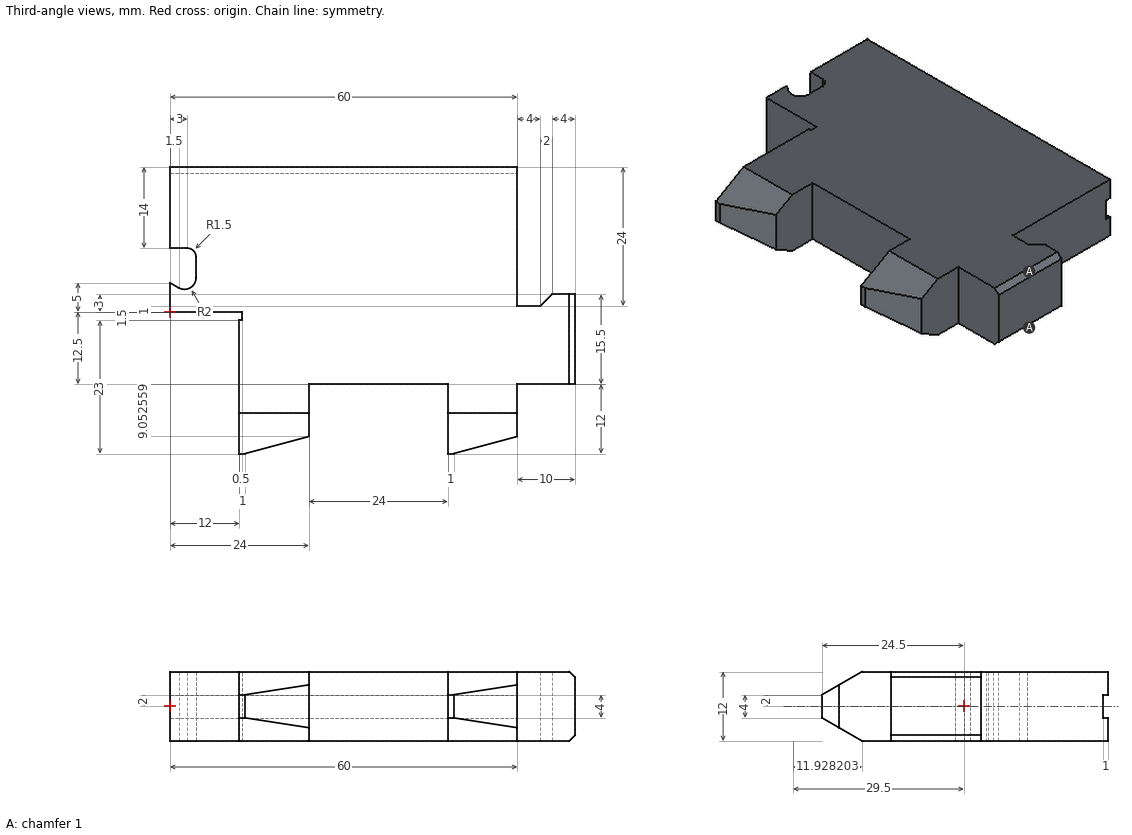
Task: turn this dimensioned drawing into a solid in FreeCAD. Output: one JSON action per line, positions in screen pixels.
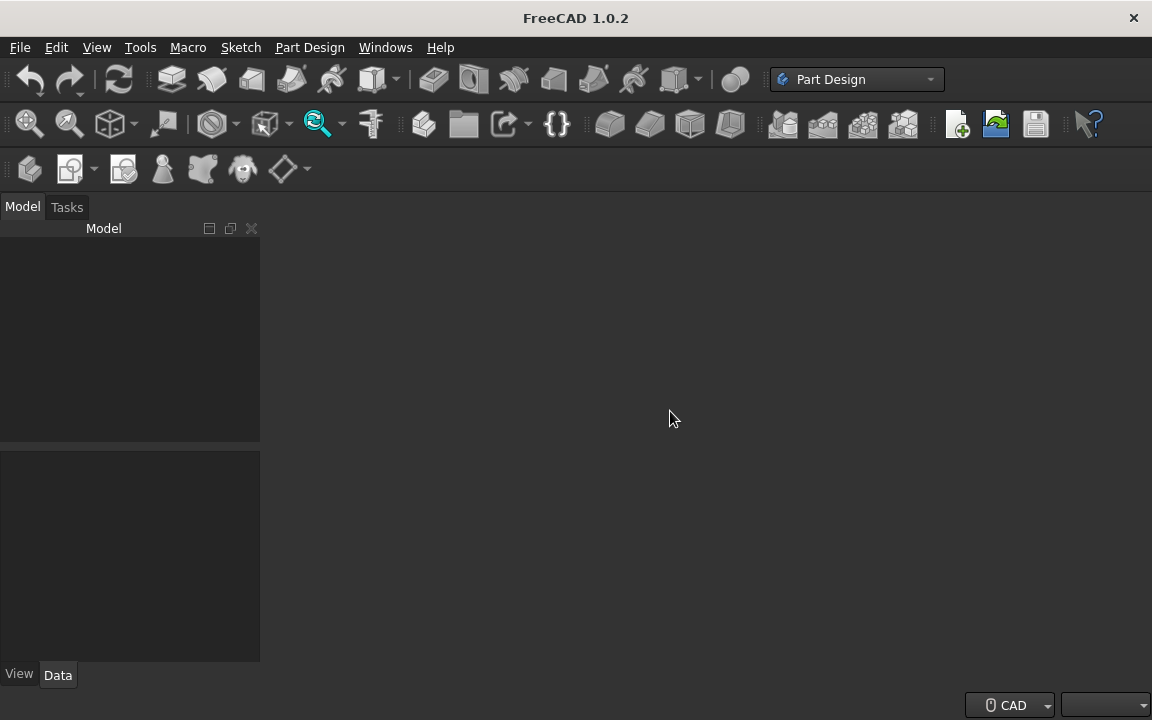
{"action": "left_click", "coordinate": [956, 124]}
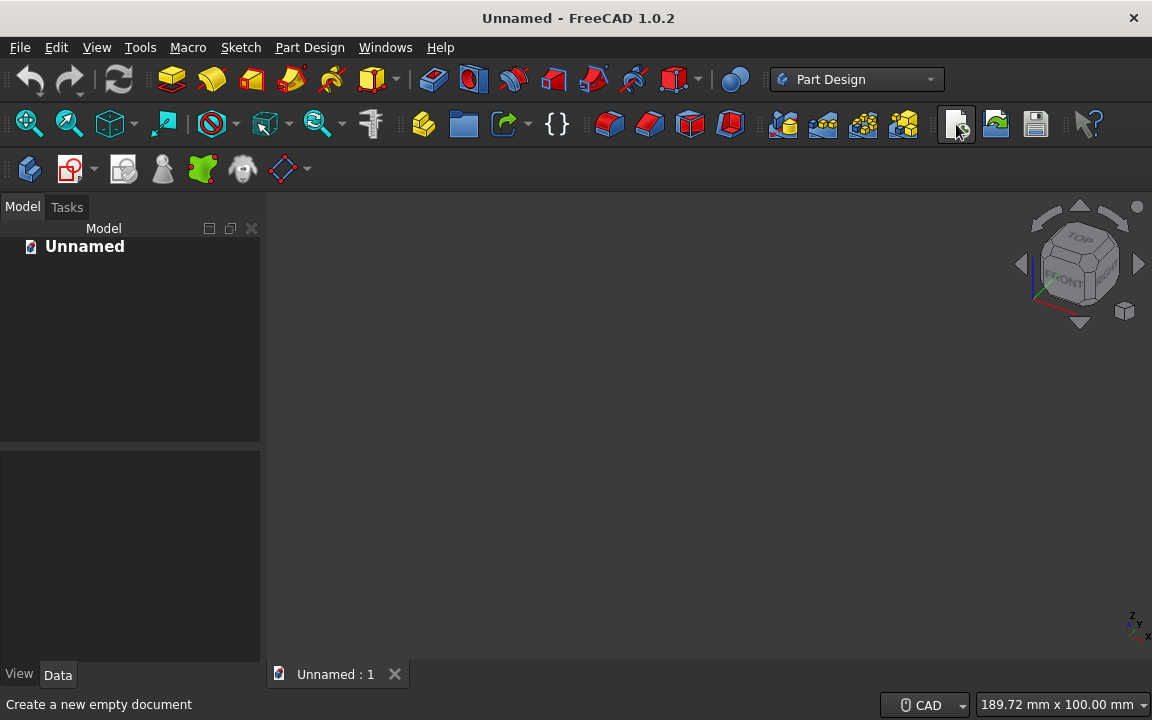
{"action": "left_click", "coordinate": [70, 170]}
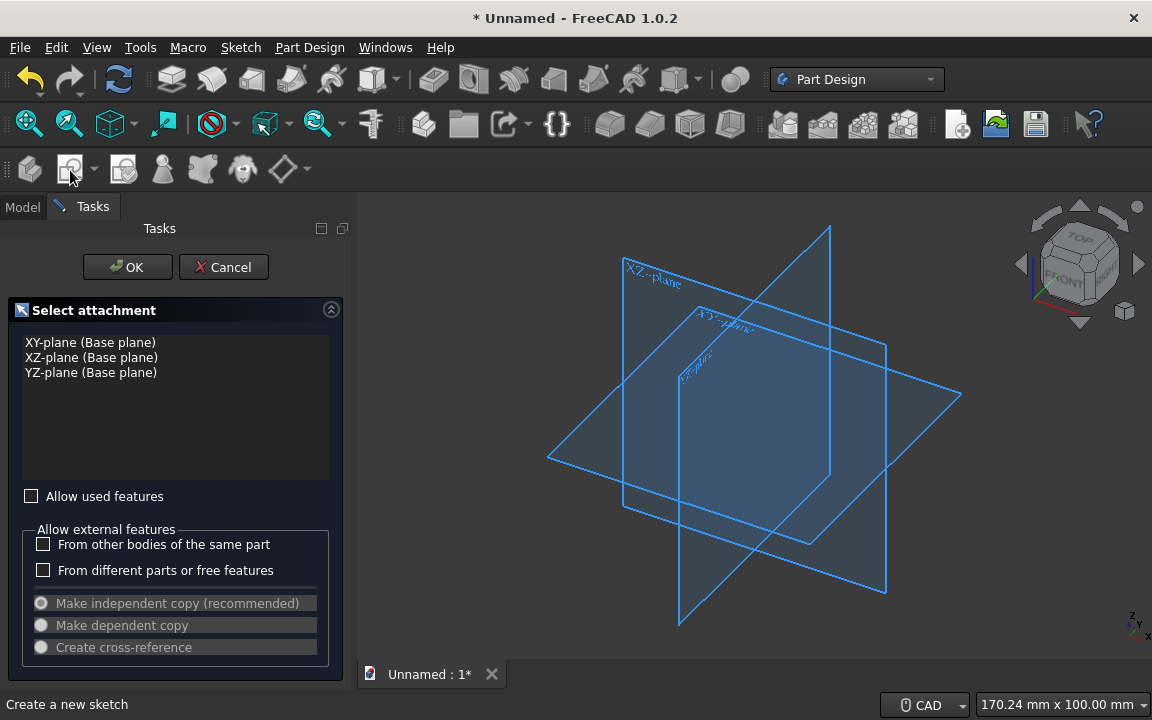
{"action": "left_click", "coordinate": [82, 342]}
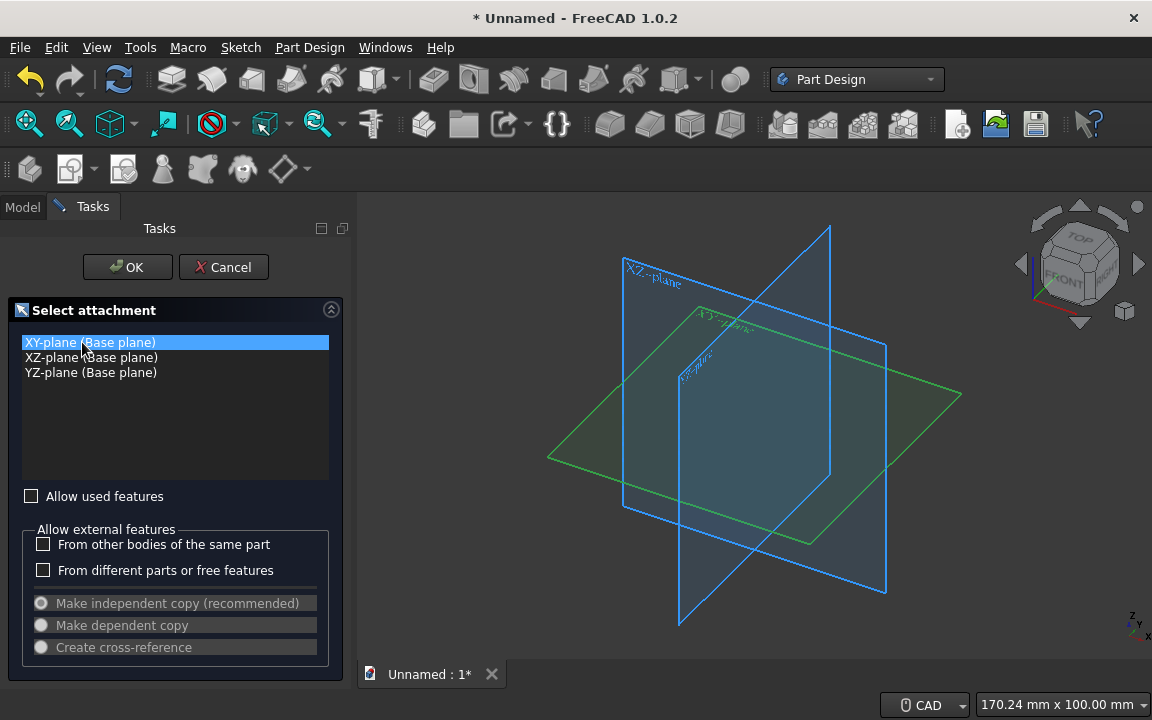
{"action": "left_click", "coordinate": [128, 267]}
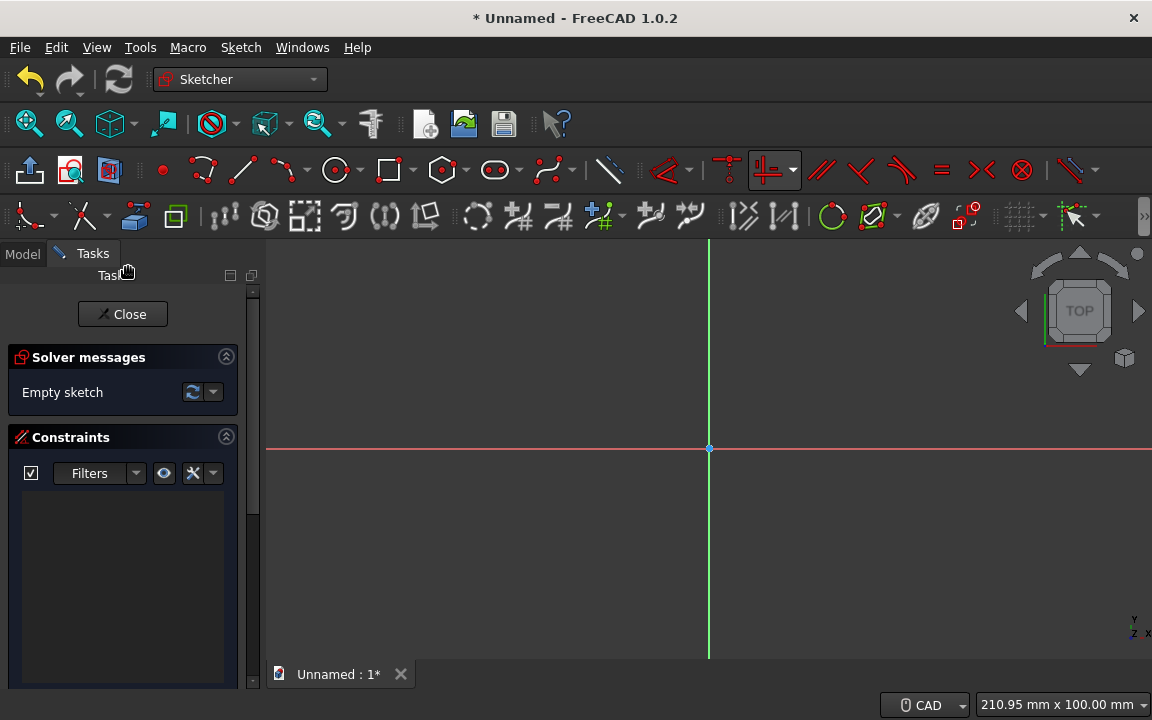
{"action": "scroll", "coordinate": [294, 454], "scroll_direction": "down", "scroll_amount": 1}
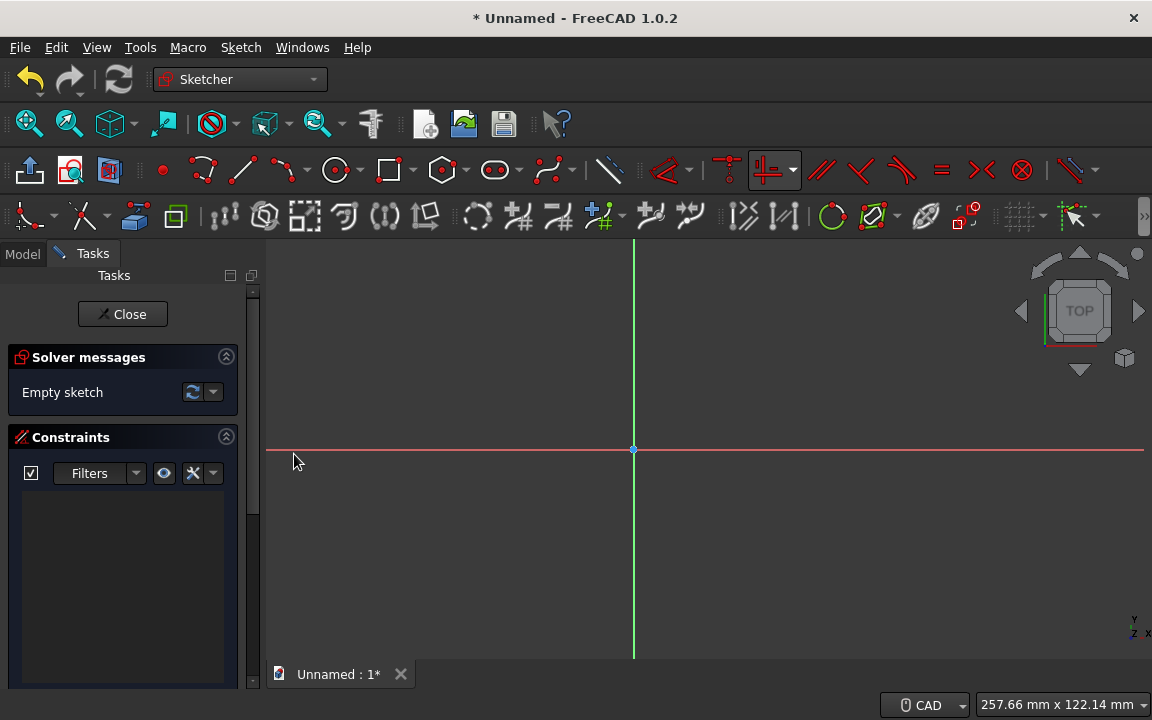
{"action": "scroll", "coordinate": [985, 449], "scroll_direction": "up", "scroll_amount": 2}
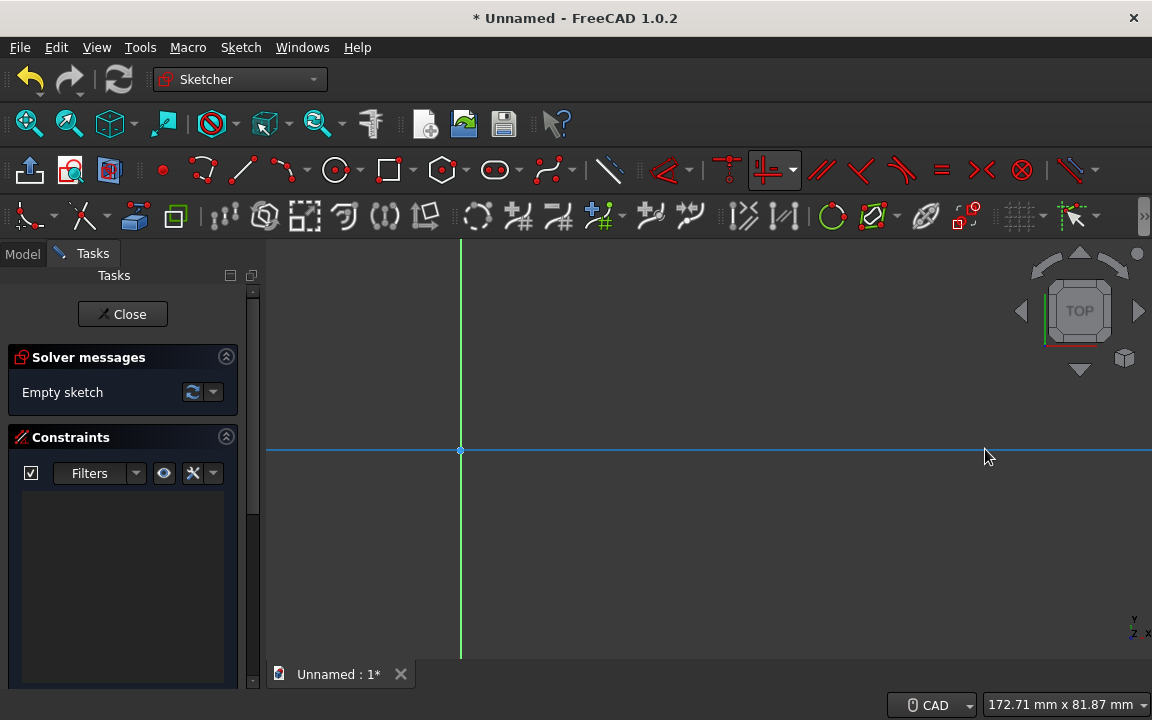
{"action": "left_click", "coordinate": [244, 170]}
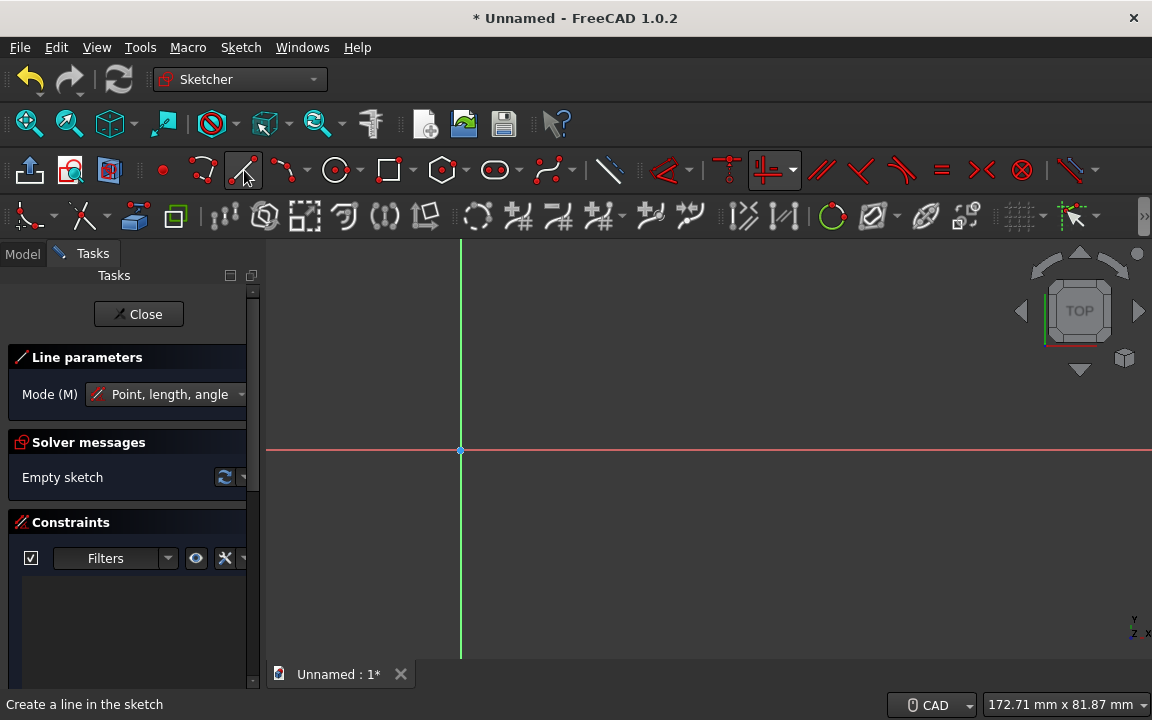
{"action": "left_click", "coordinate": [484, 402]}
{"action": "left_click", "coordinate": [484, 420]}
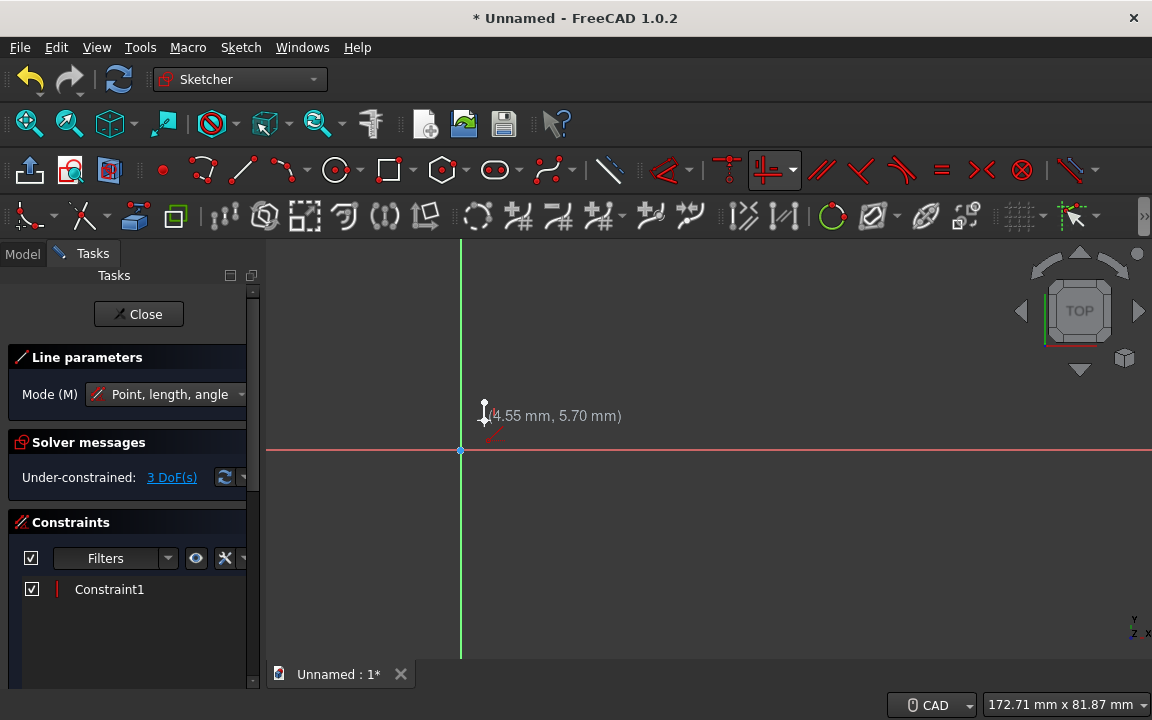
{"action": "left_click", "coordinate": [204, 170]}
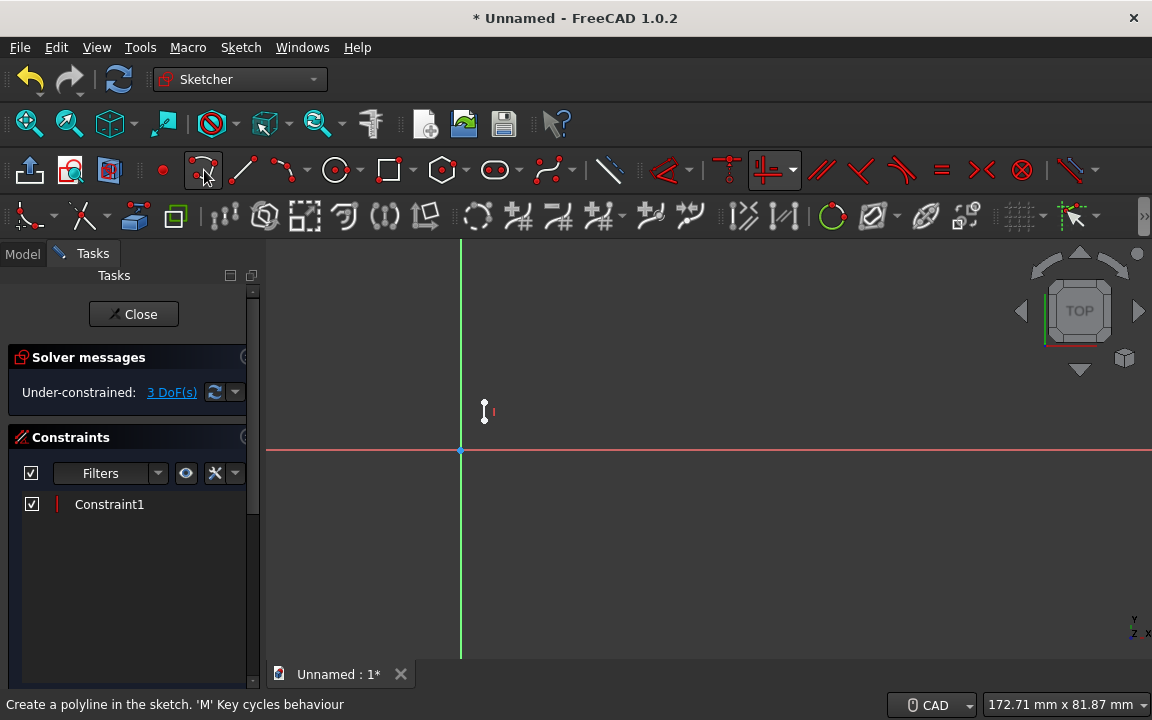
{"action": "scroll", "coordinate": [468, 429], "scroll_direction": "up", "scroll_amount": 4}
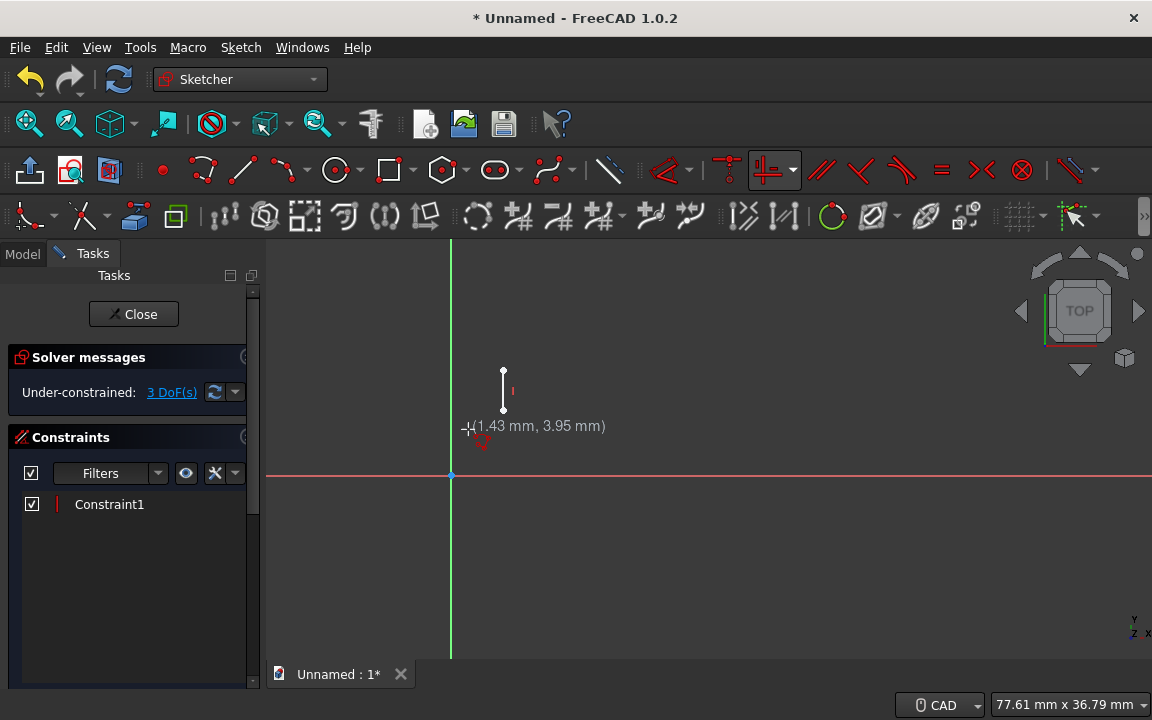
{"action": "left_click", "coordinate": [468, 429]}
{"action": "left_click", "coordinate": [451, 419]}
{"action": "left_click", "coordinate": [451, 476]}
{"action": "left_click", "coordinate": [594, 467]}
{"action": "left_click", "coordinate": [594, 493]}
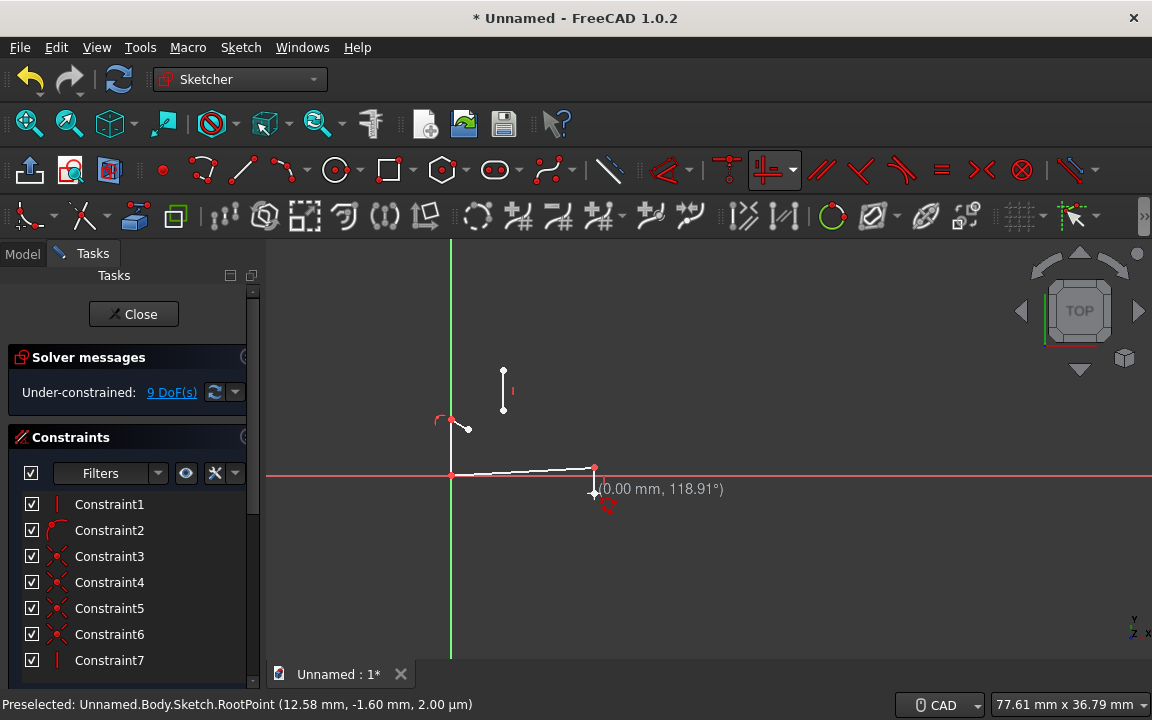
{"action": "scroll", "coordinate": [588, 493], "scroll_direction": "up", "scroll_amount": 6}